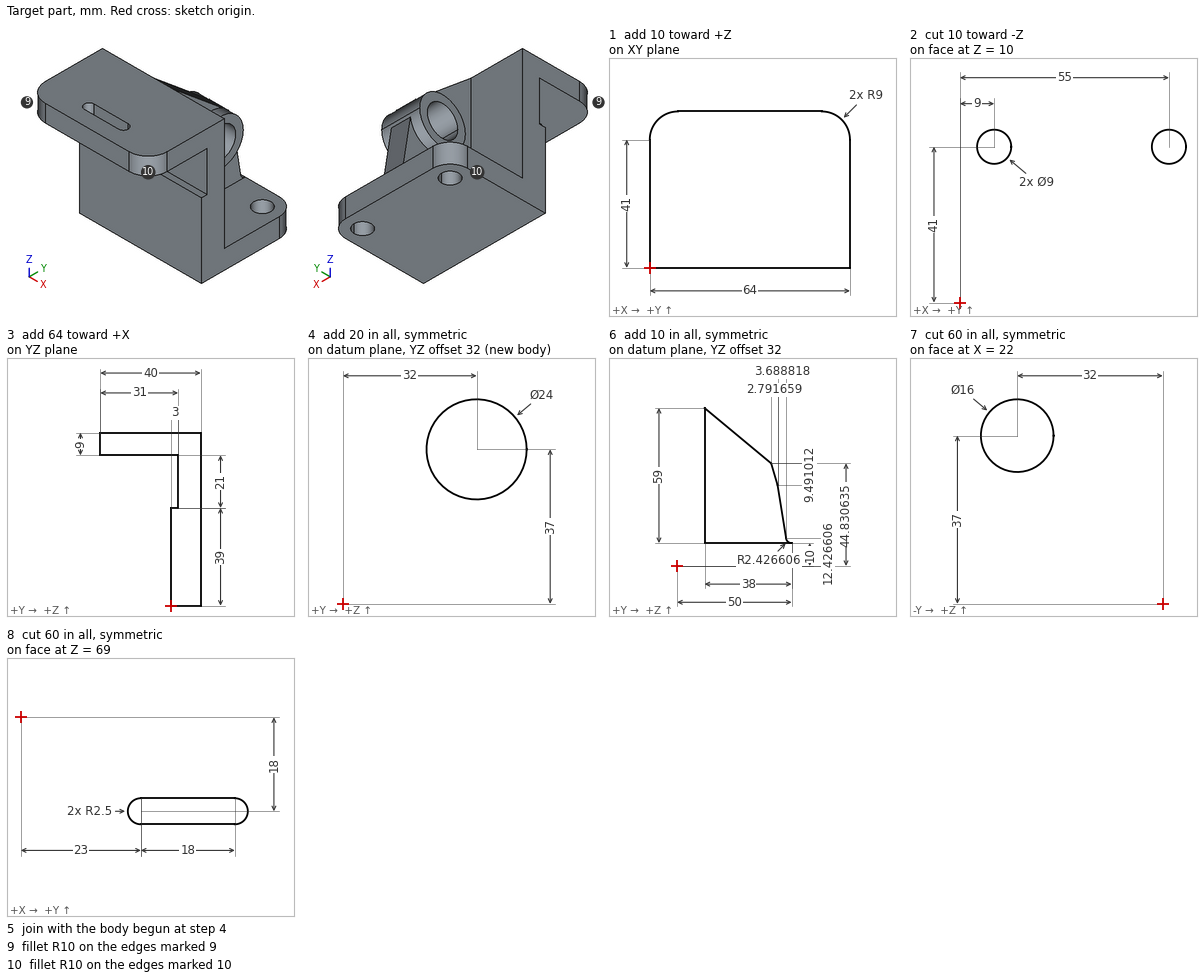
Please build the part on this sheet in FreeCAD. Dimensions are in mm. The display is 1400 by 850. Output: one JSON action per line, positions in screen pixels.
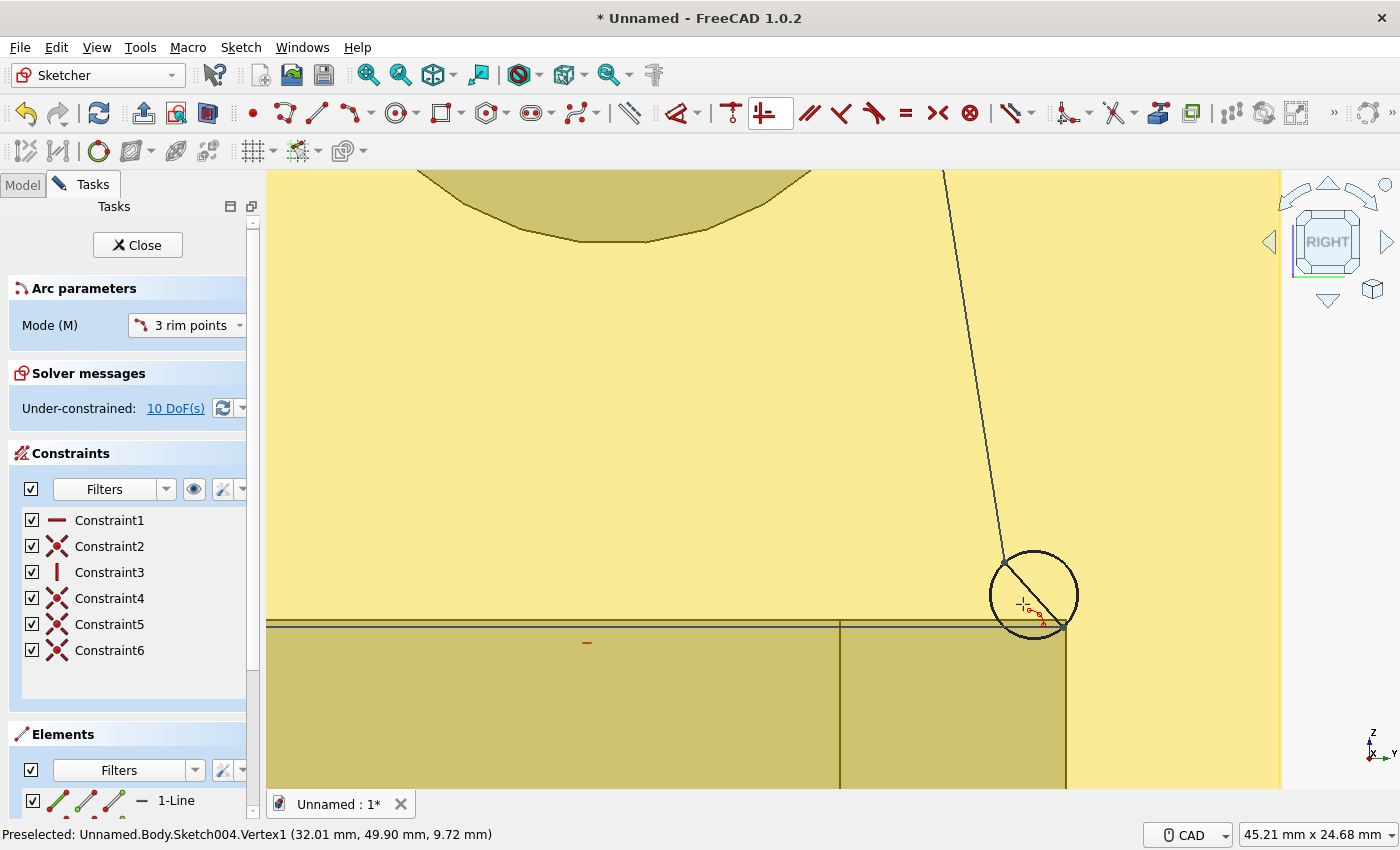
{"action": "left_click", "coordinate": [1023, 603]}
{"action": "key", "text": "Escape"}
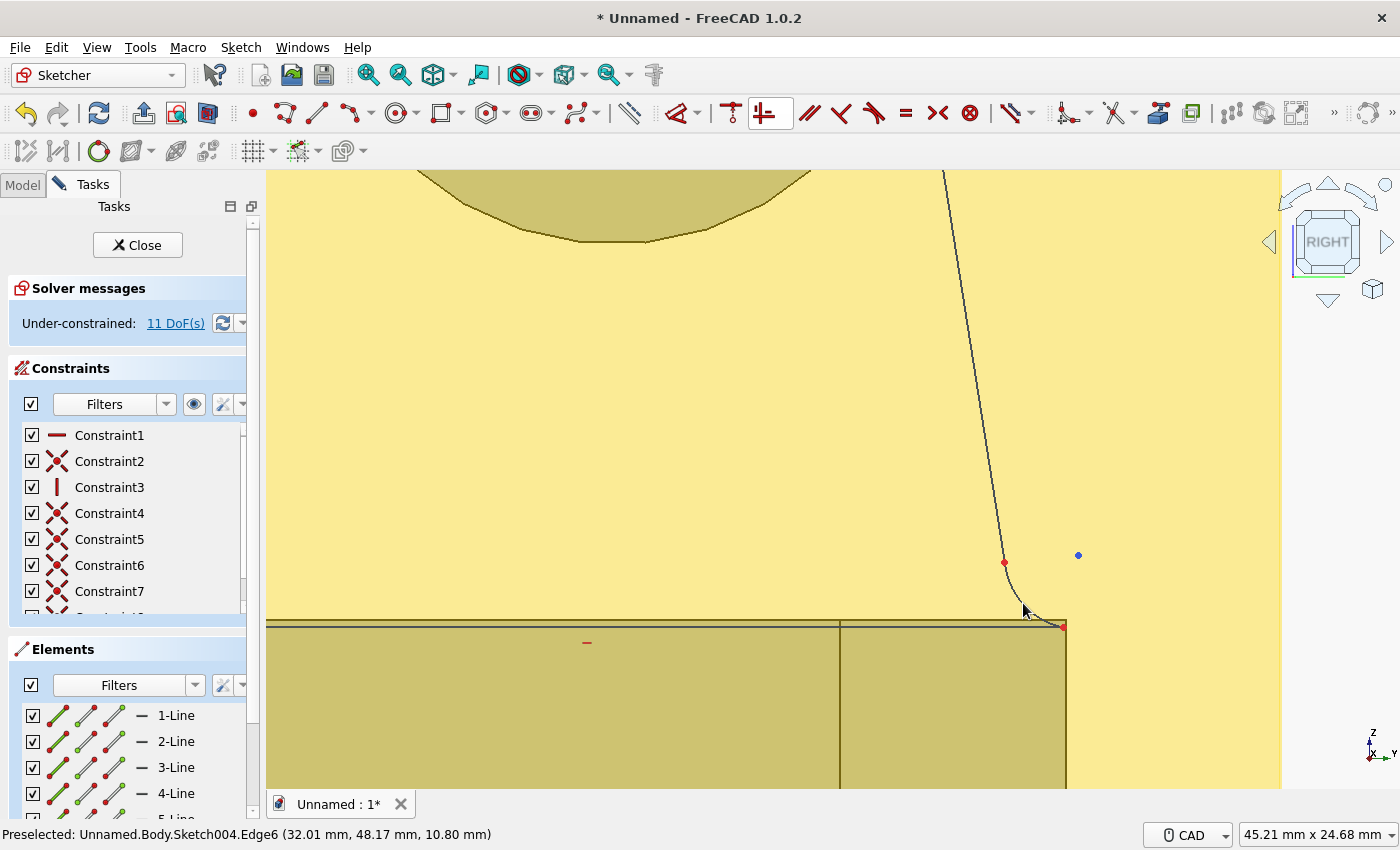
{"action": "scroll", "coordinate": [871, 635], "scroll_direction": "down", "scroll_amount": 7}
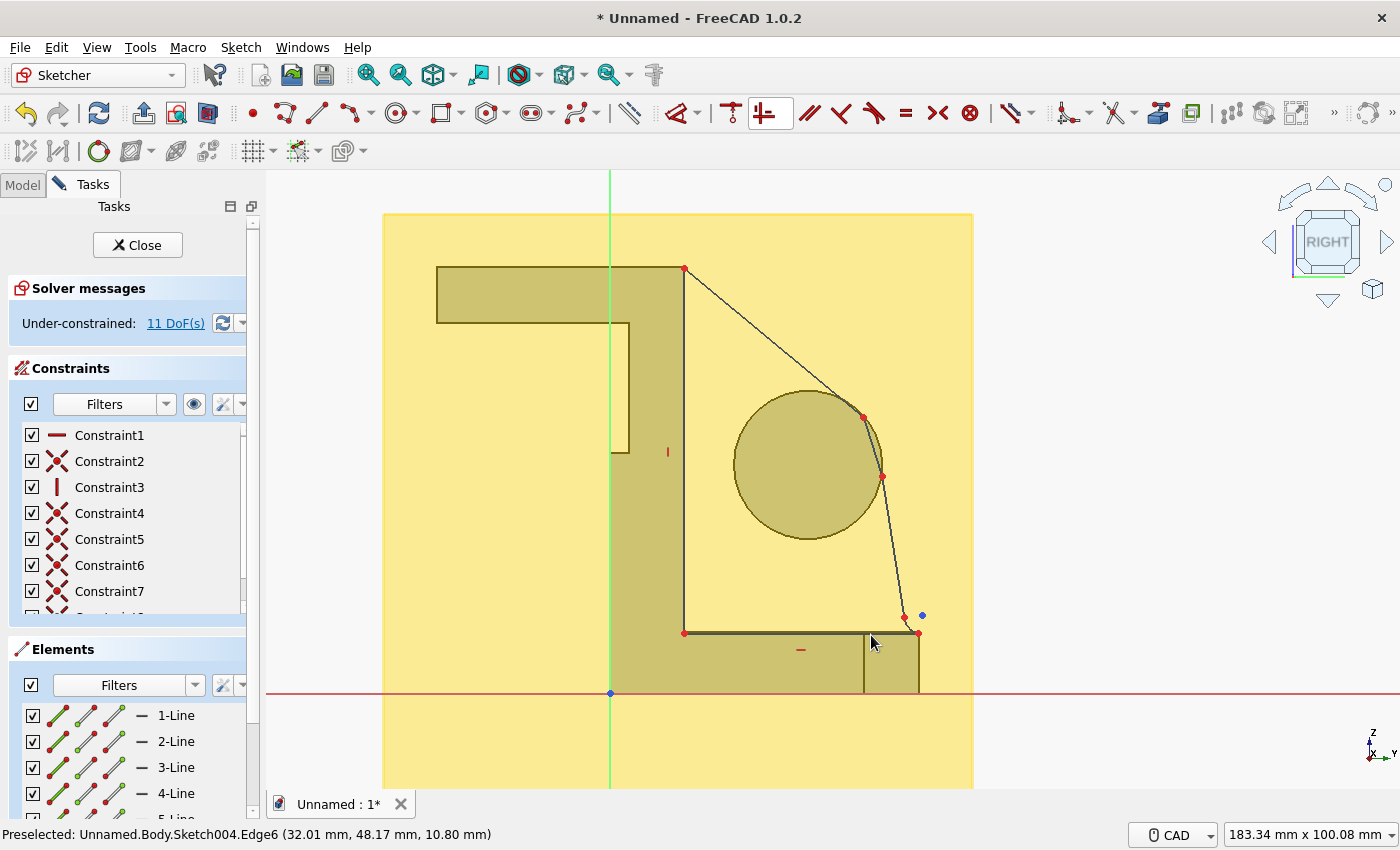
{"action": "left_click", "coordinate": [848, 634]}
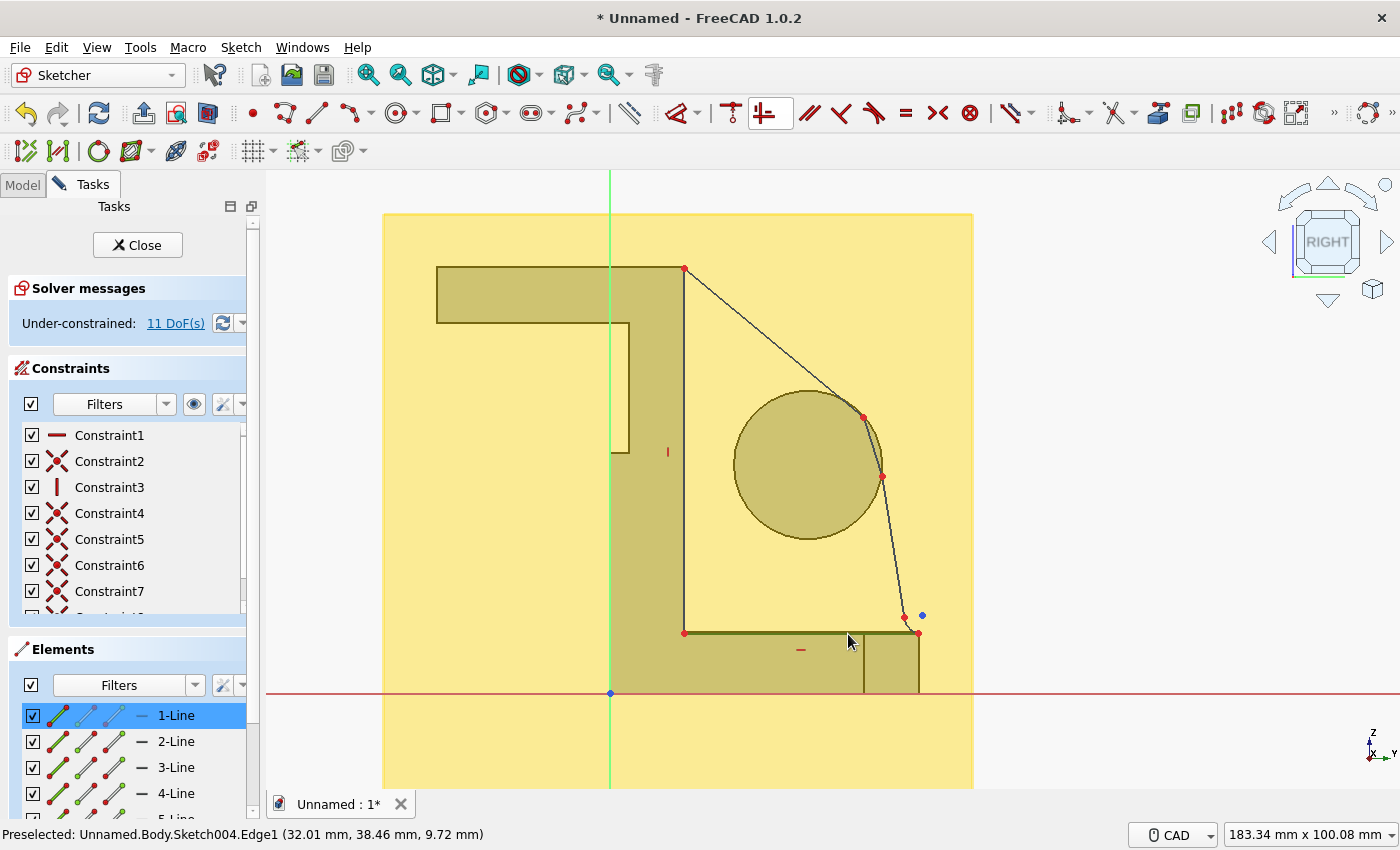
{"action": "scroll", "coordinate": [906, 624], "scroll_direction": "up", "scroll_amount": 4}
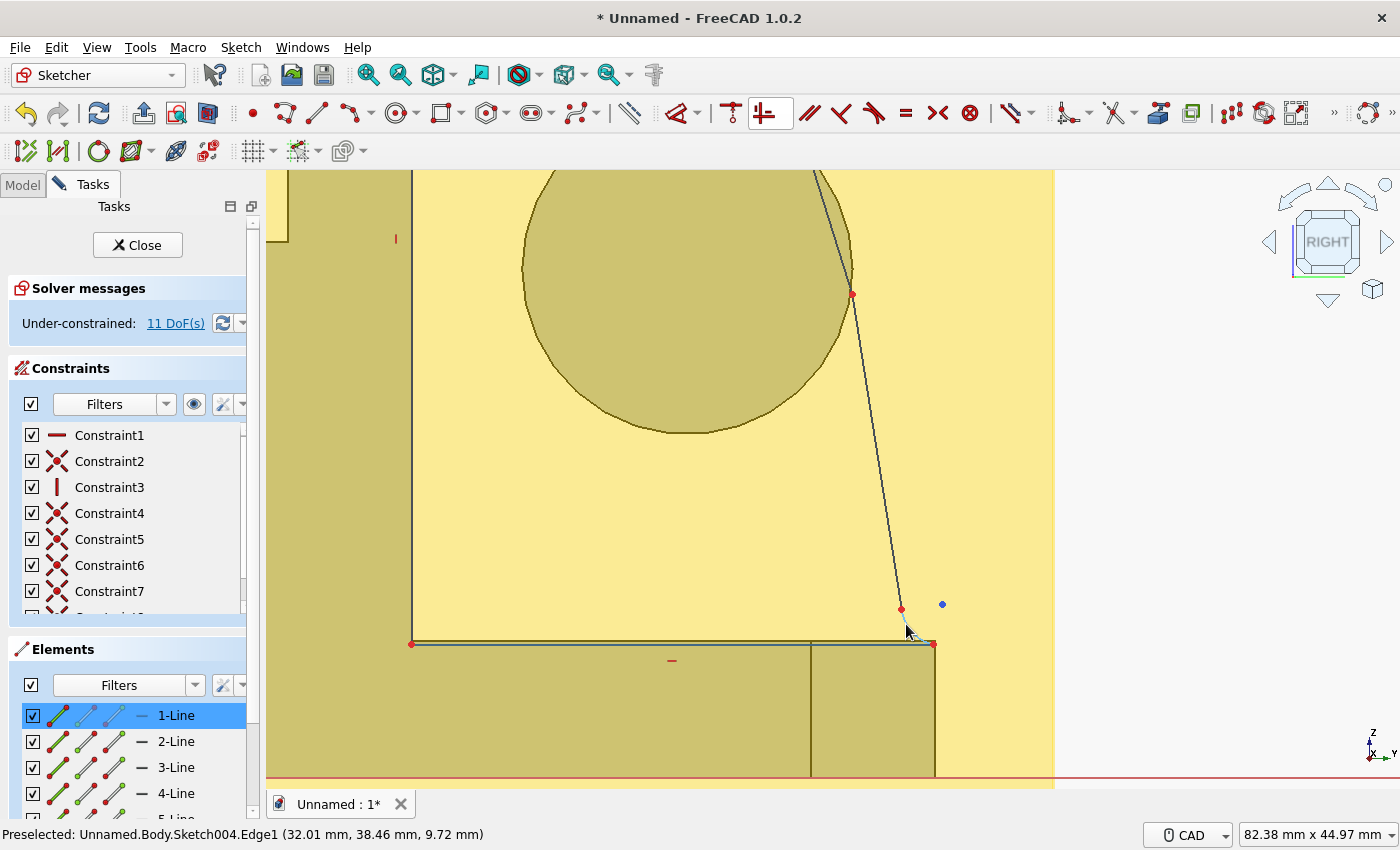
{"action": "left_click", "coordinate": [906, 624]}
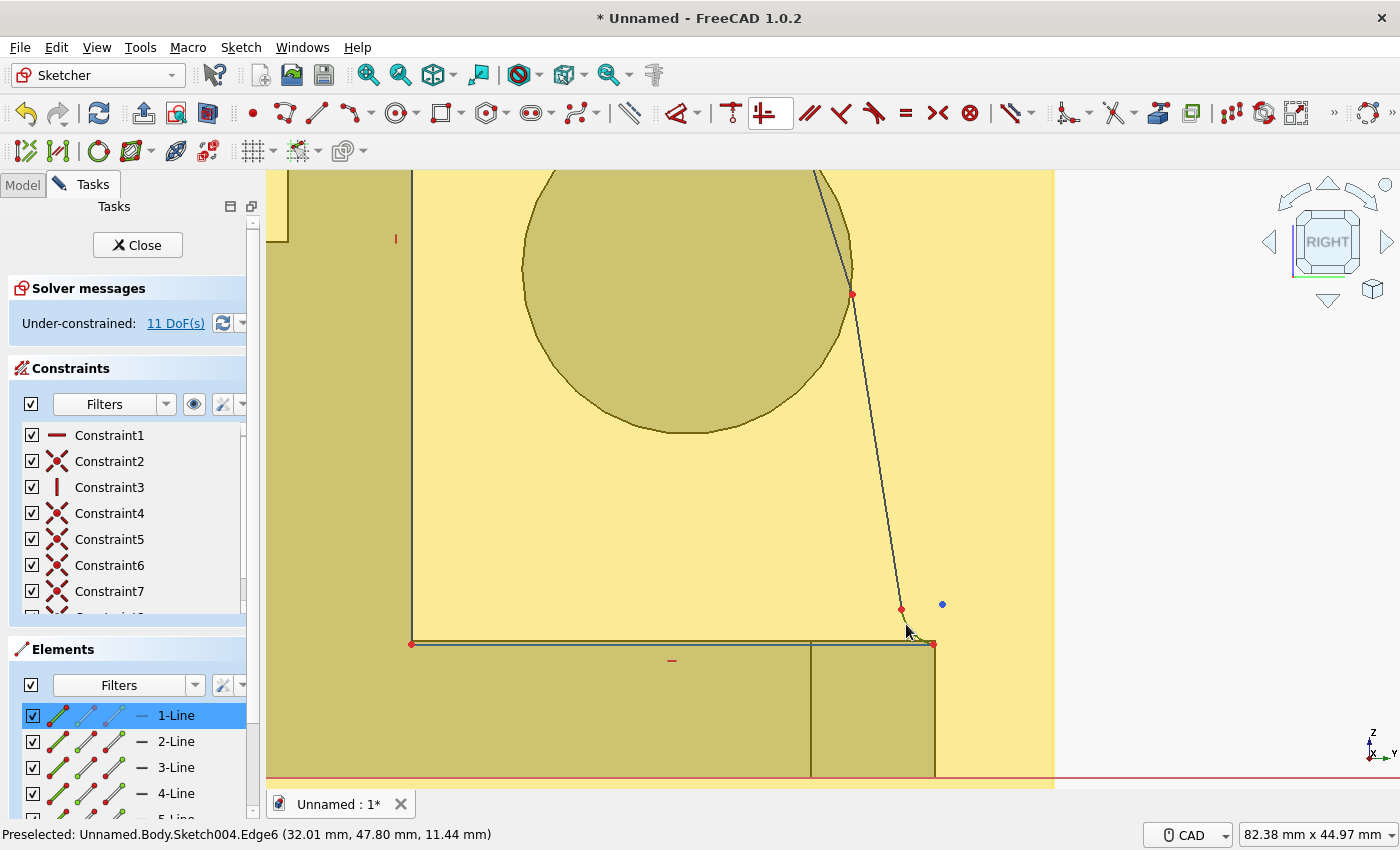
{"action": "left_click", "coordinate": [874, 114]}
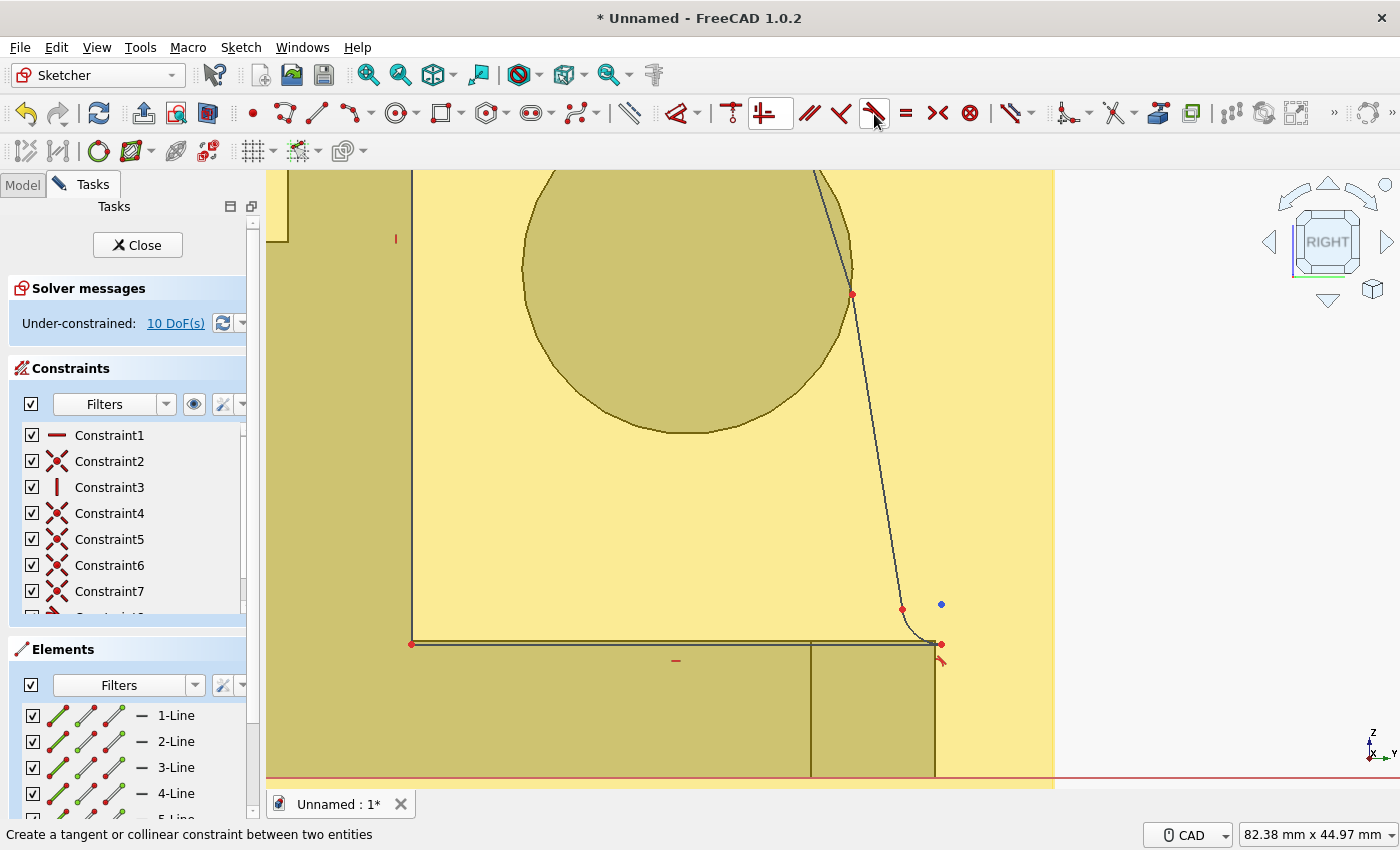
{"action": "left_click", "coordinate": [676, 114]}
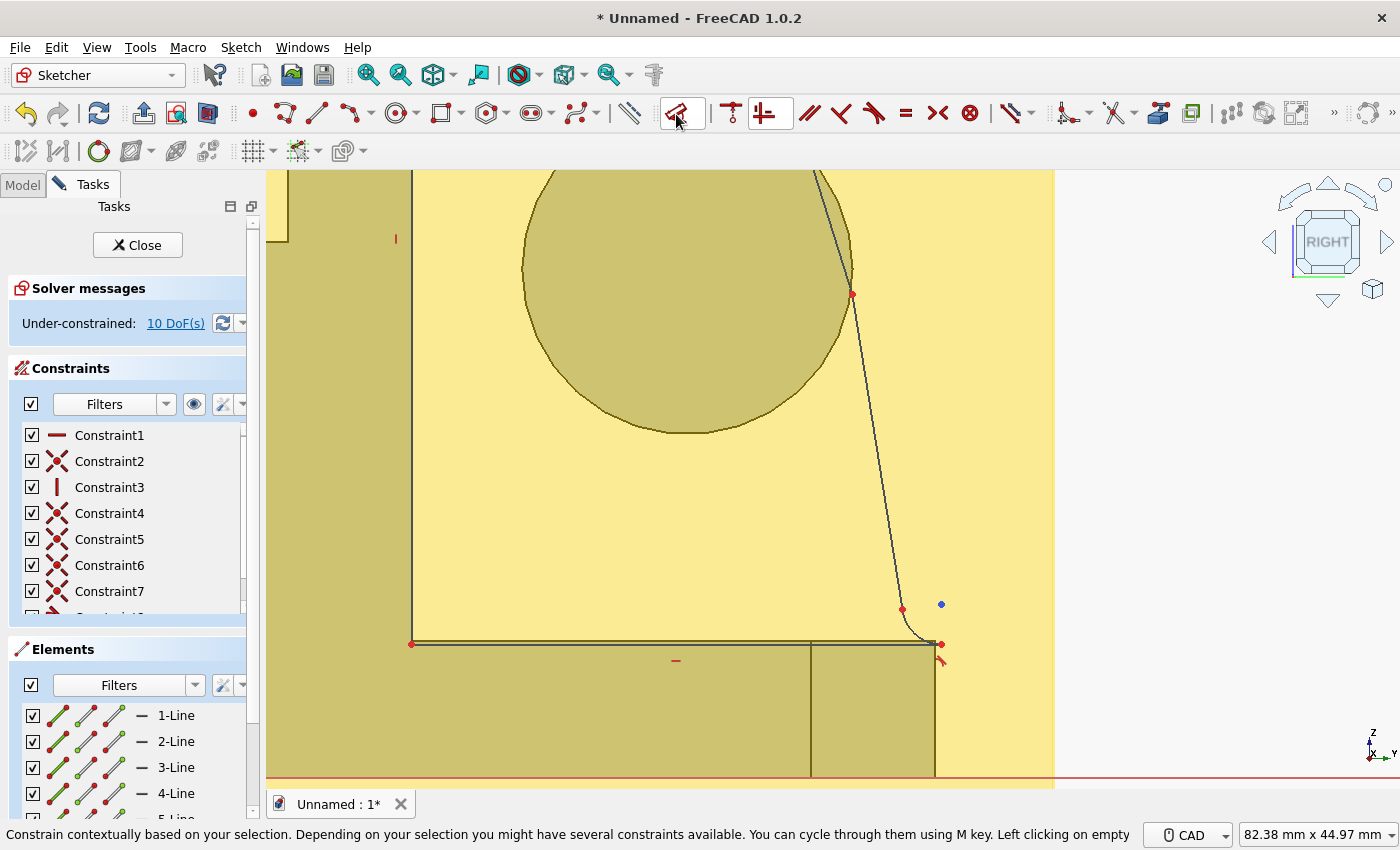
{"action": "left_click", "coordinate": [908, 625]}
{"action": "left_click", "coordinate": [871, 607]}